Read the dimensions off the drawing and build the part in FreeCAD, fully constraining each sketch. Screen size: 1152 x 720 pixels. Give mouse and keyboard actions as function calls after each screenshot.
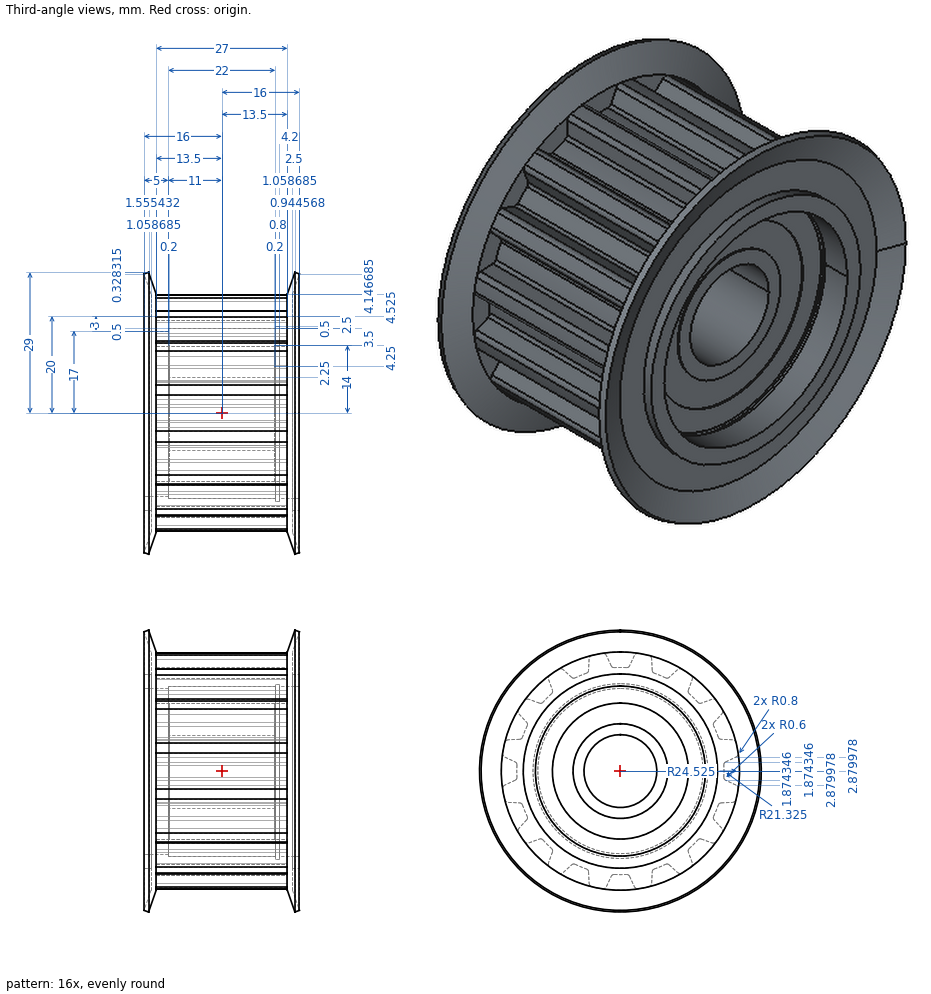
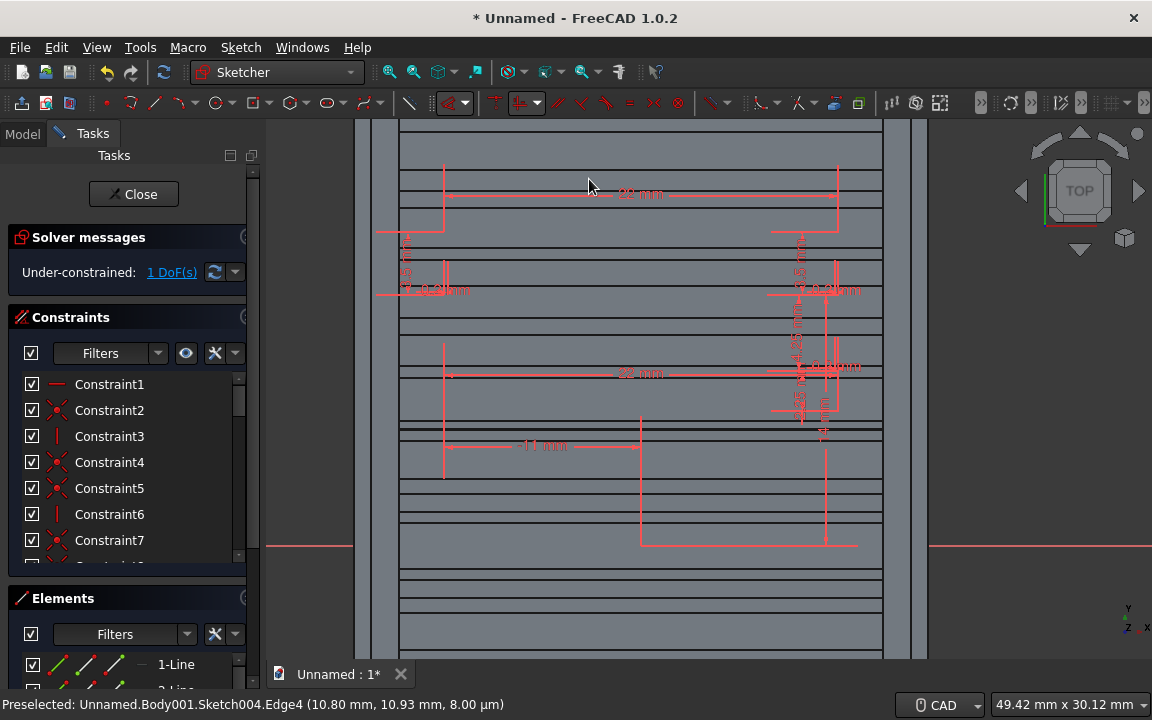
click(448, 318)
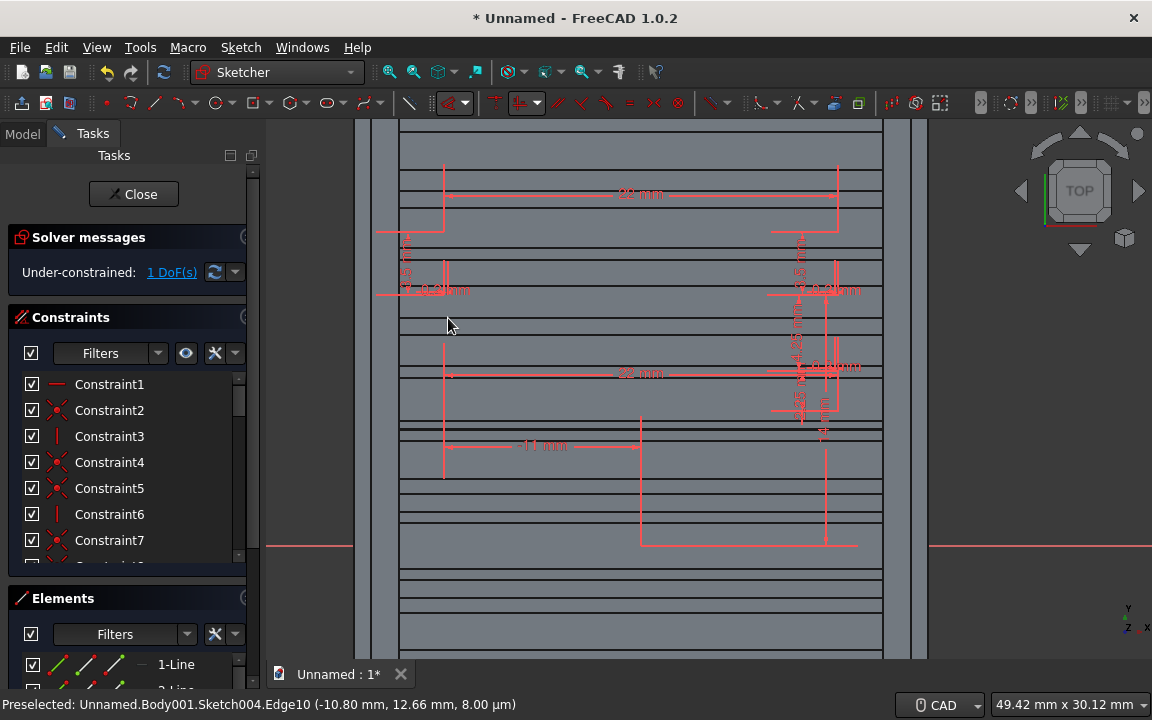
click(468, 104)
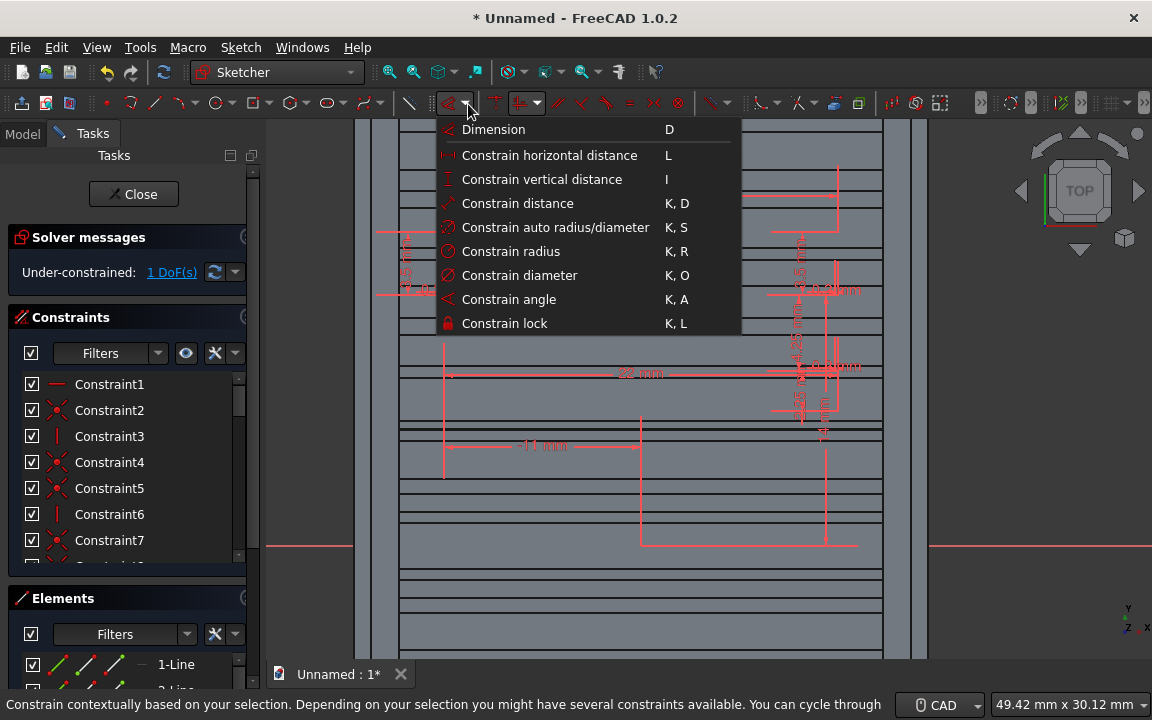
click(589, 179)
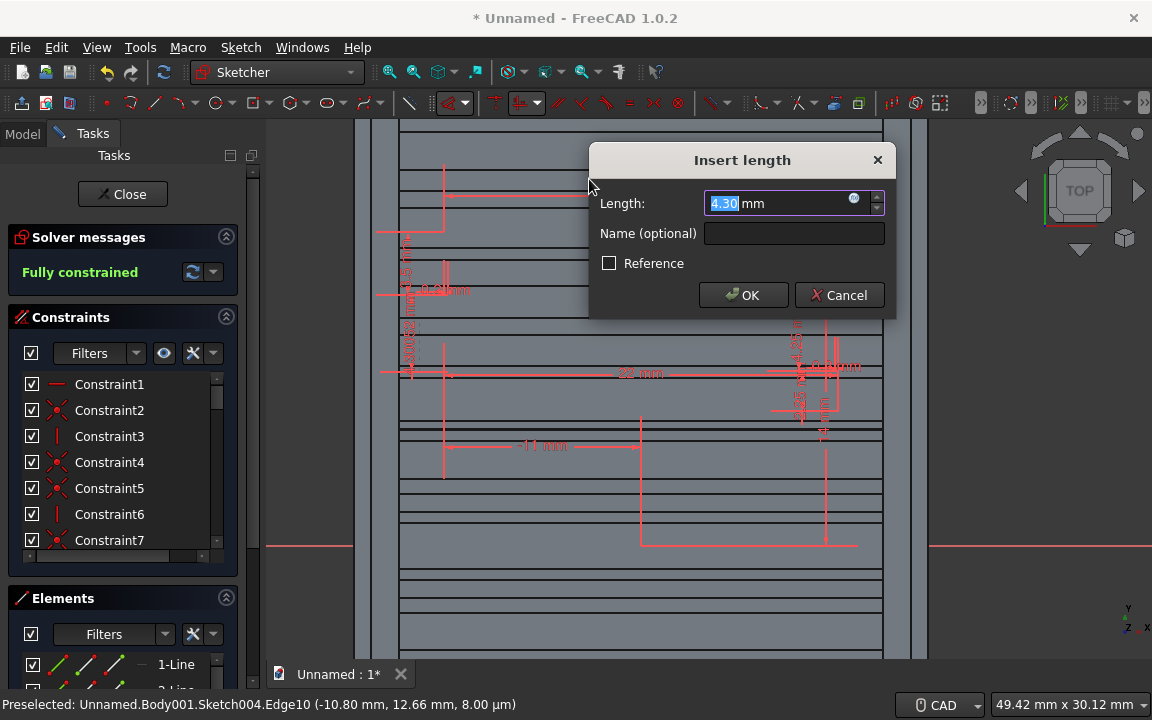
text(4.25)
key(Return)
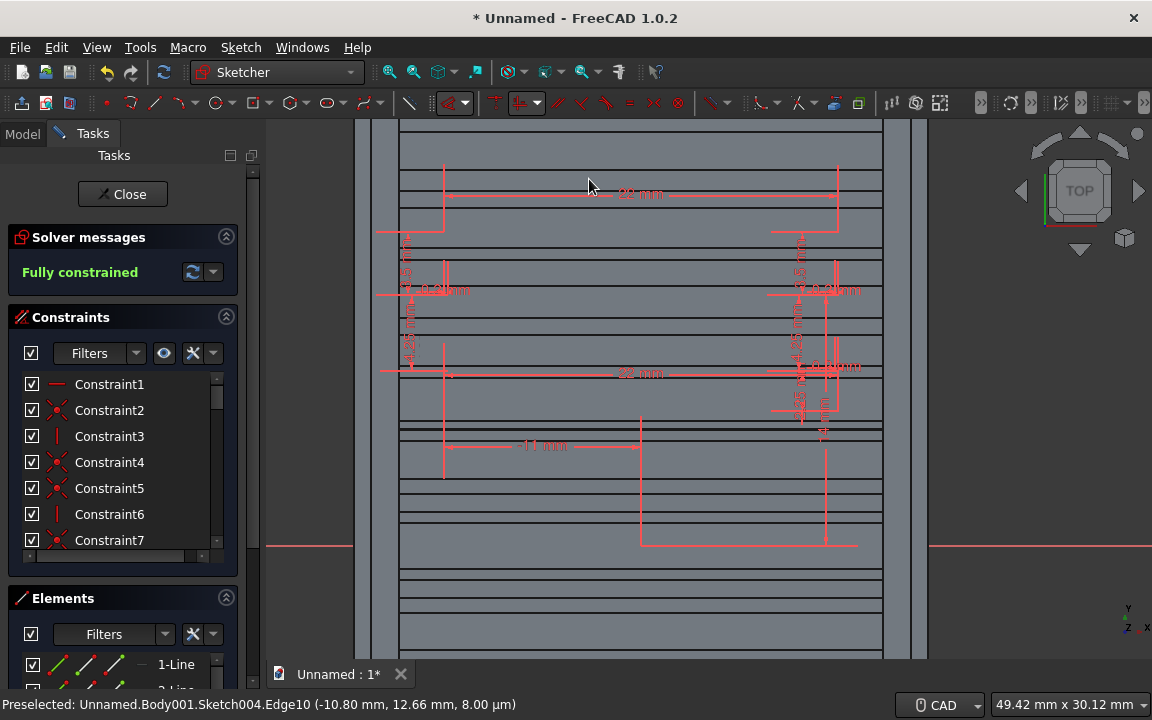
click(123, 194)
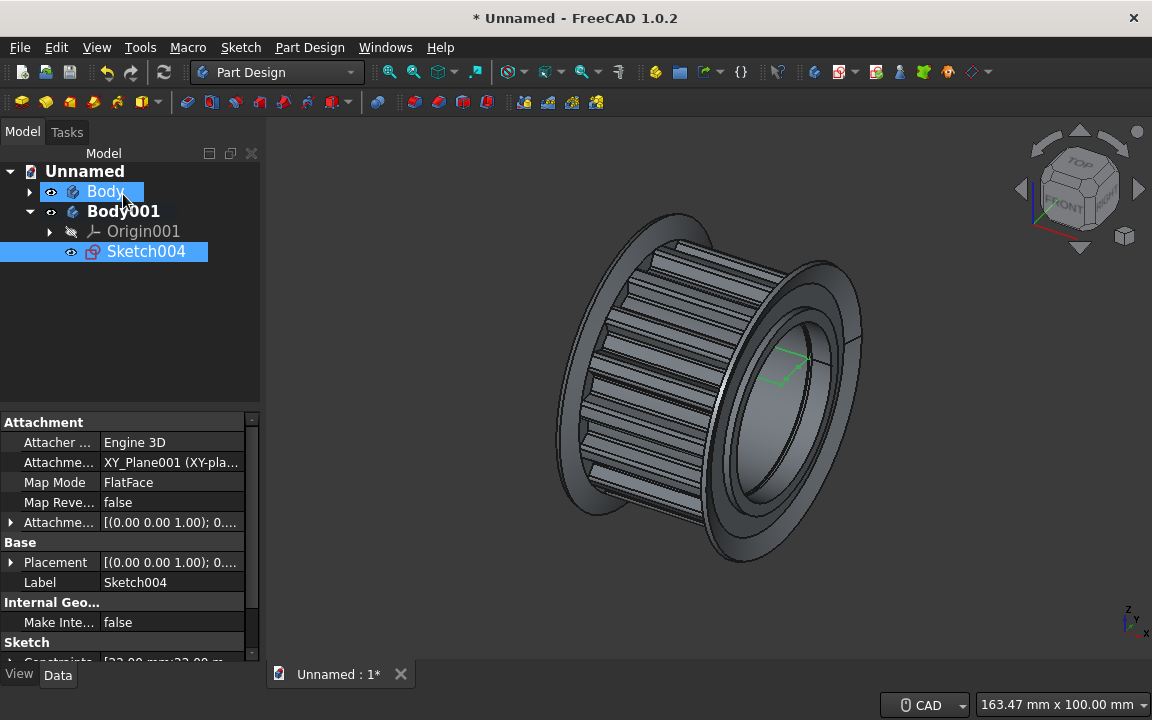
click(46, 102)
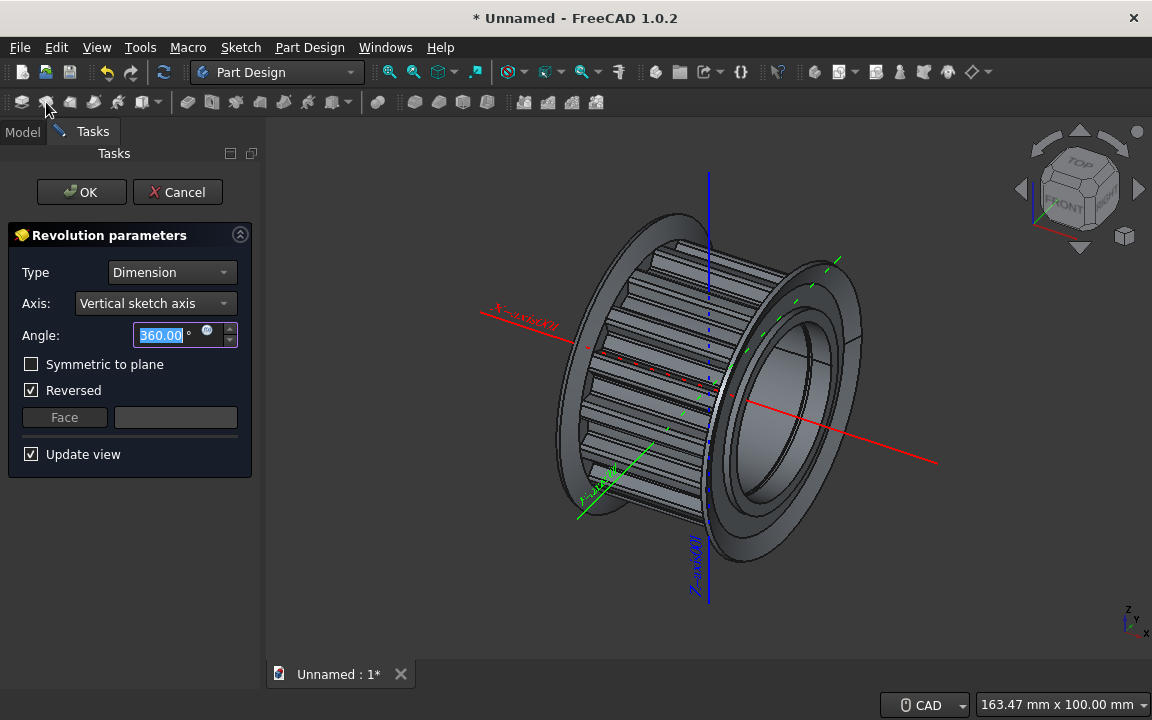
click(156, 304)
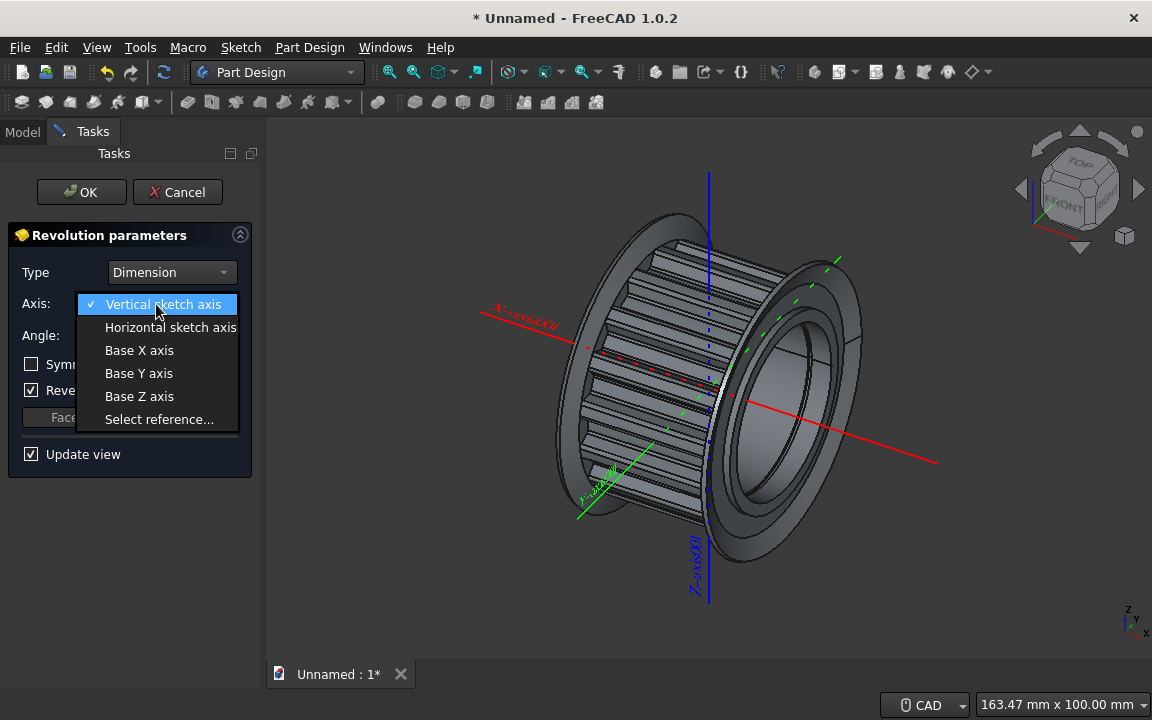
click(156, 328)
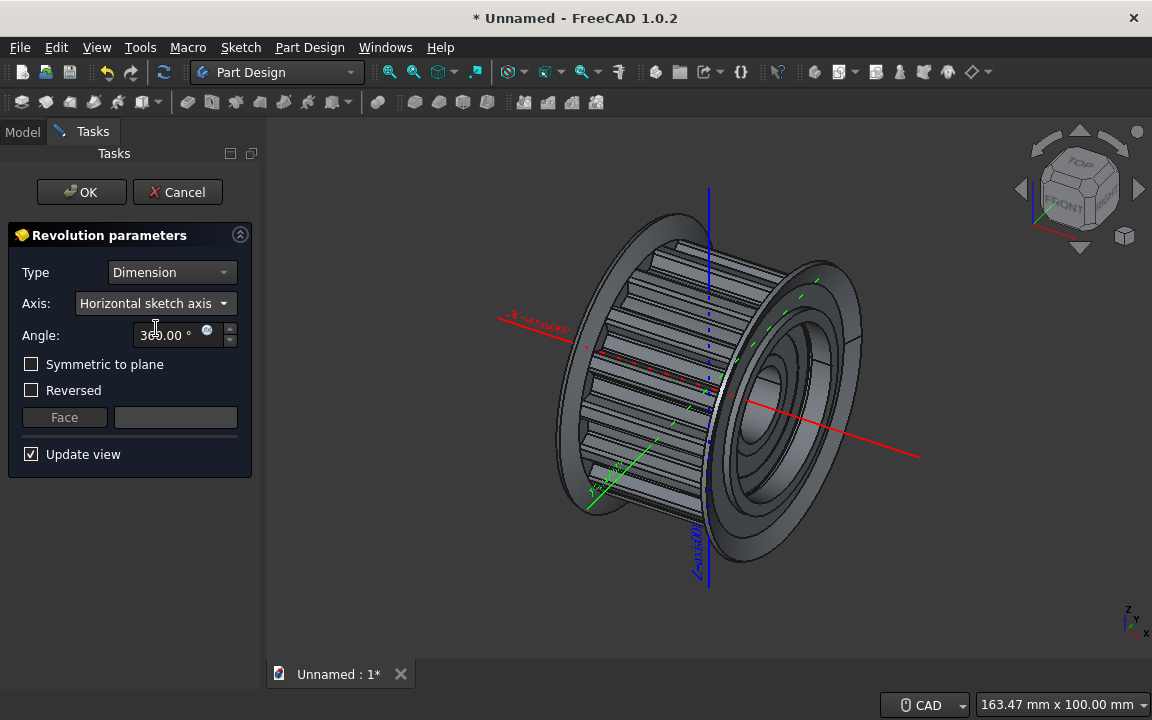
click(82, 192)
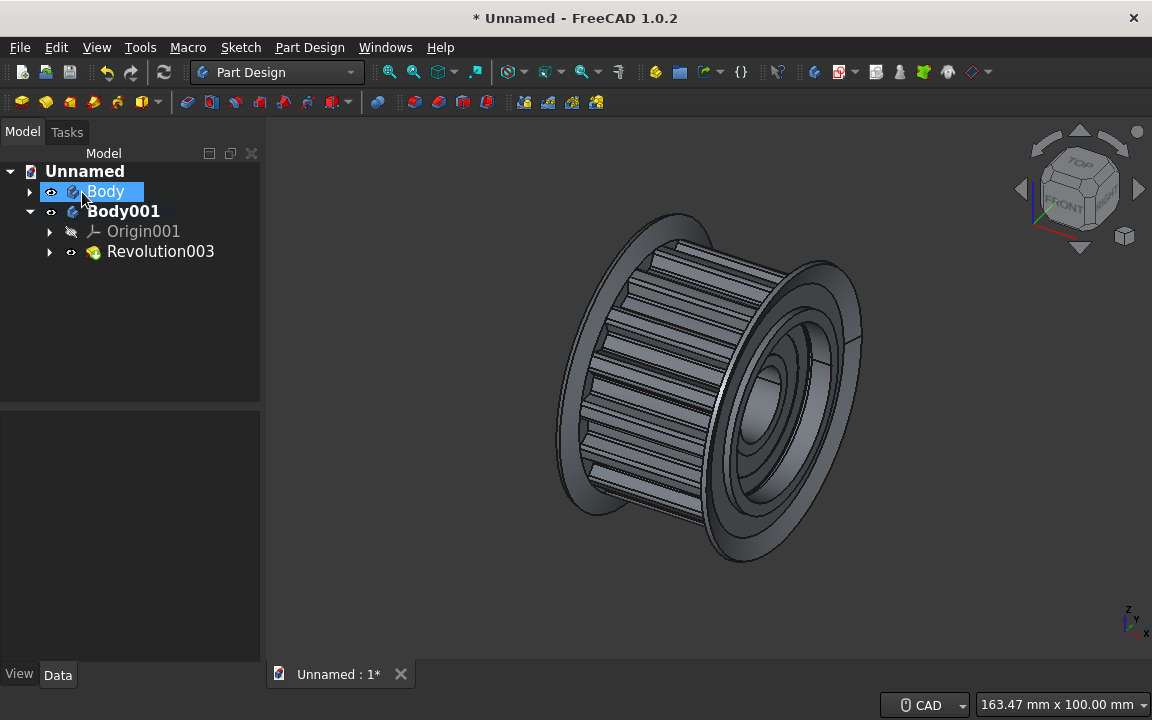
key(0)